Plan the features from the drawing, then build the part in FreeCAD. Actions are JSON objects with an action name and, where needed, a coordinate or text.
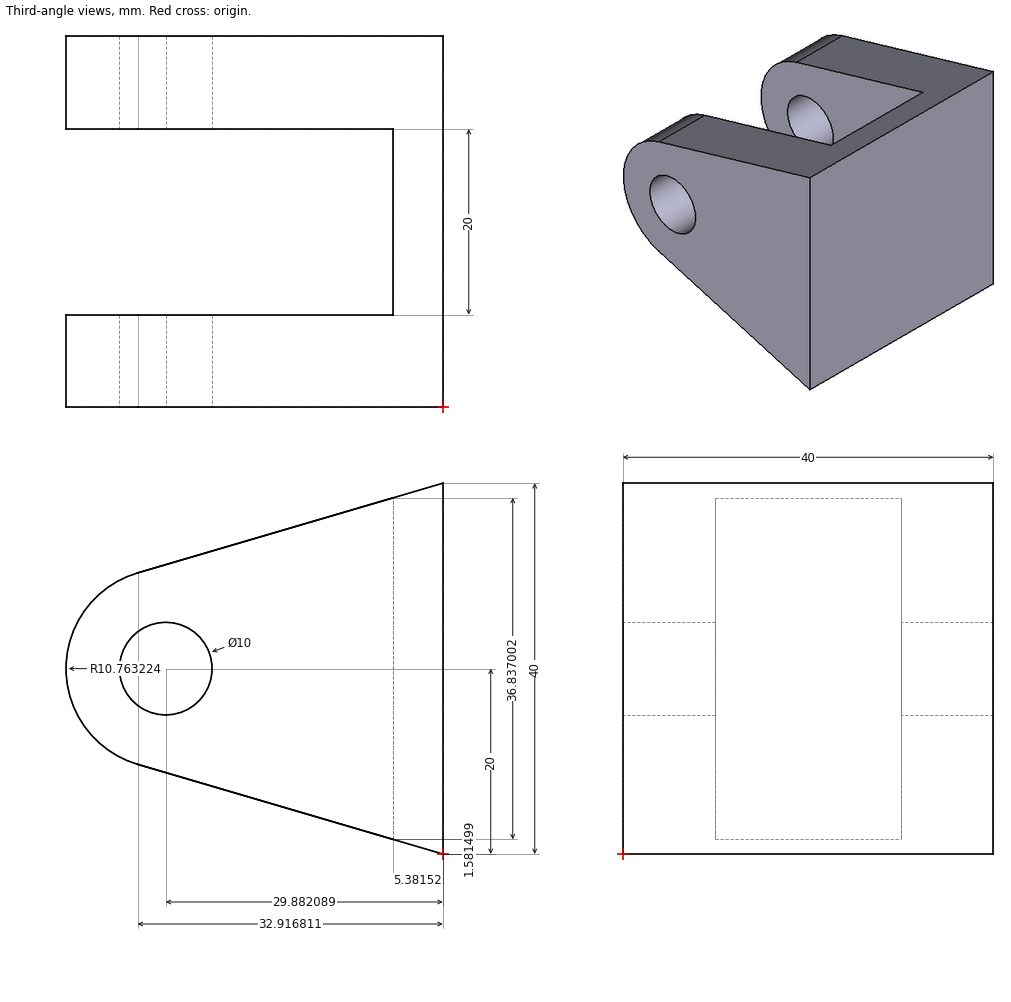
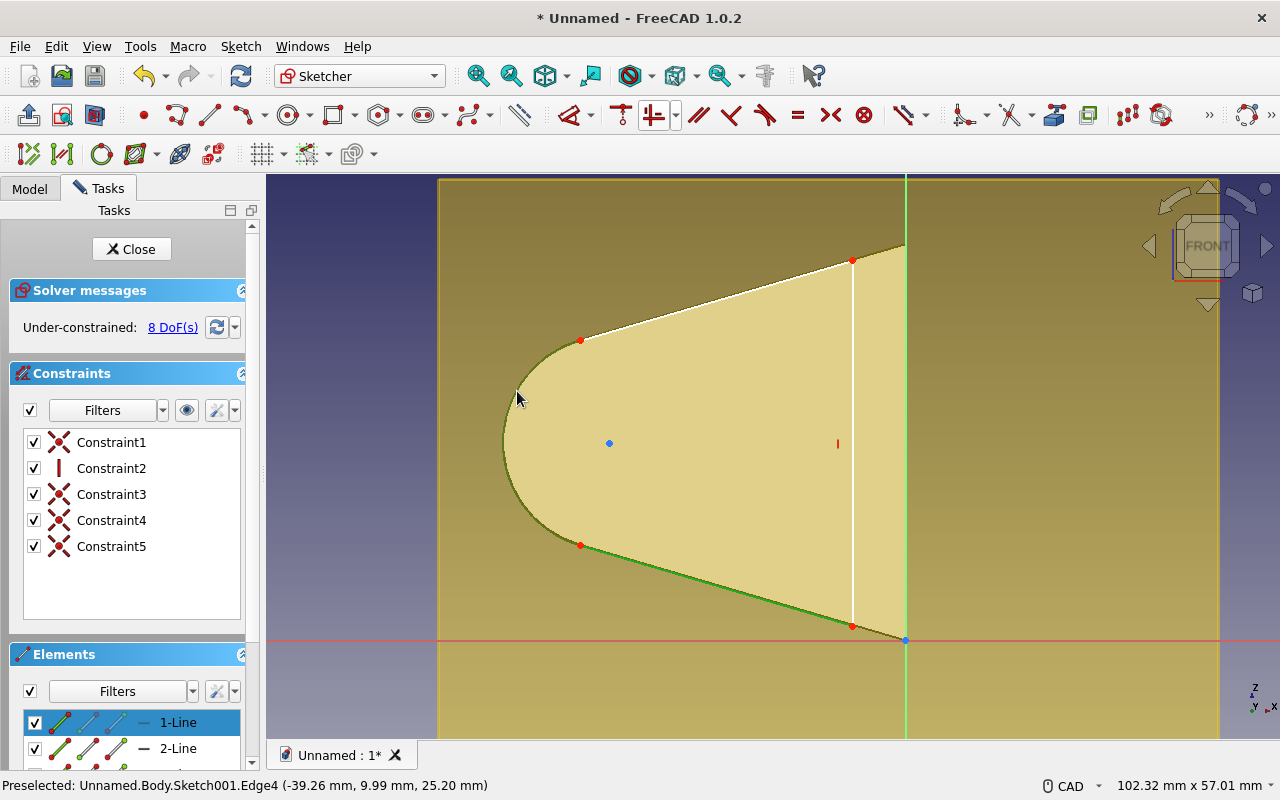
{"action": "left_click", "coordinate": [765, 116]}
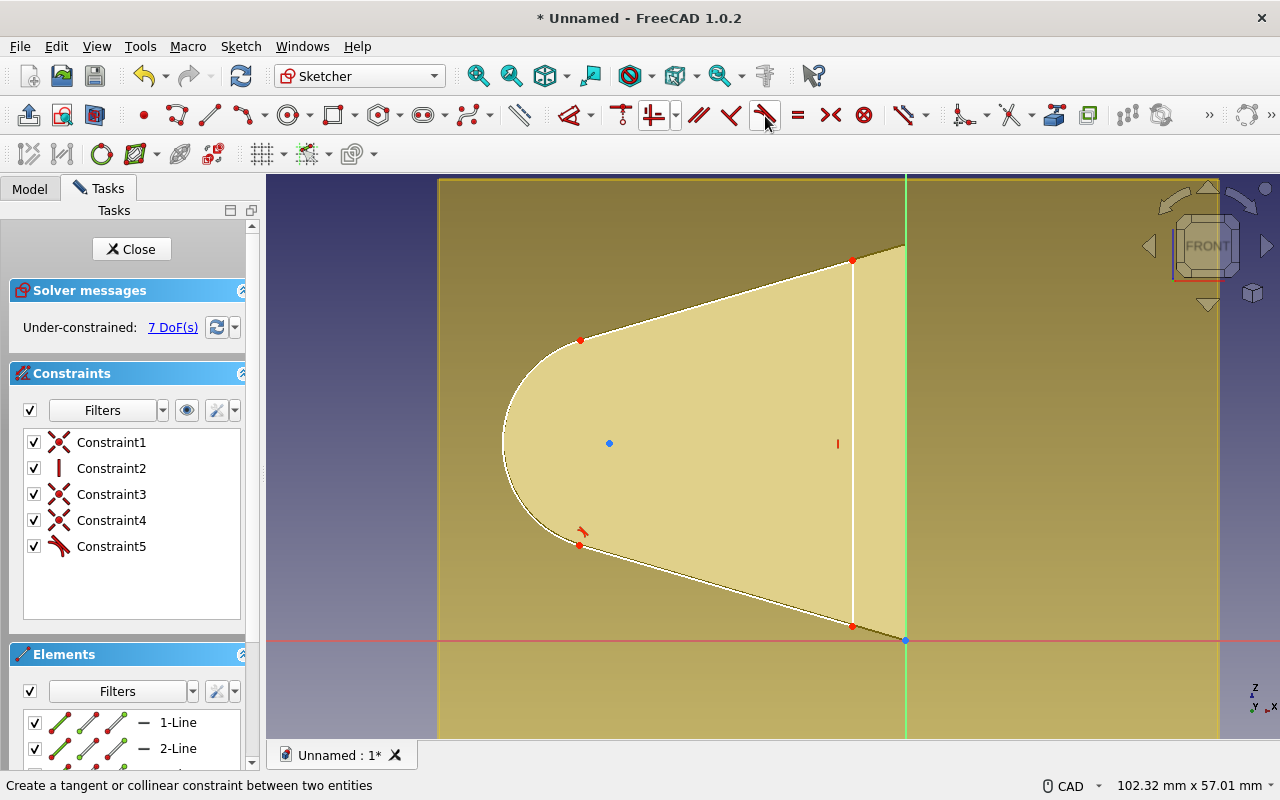
{"action": "left_click", "coordinate": [771, 285]}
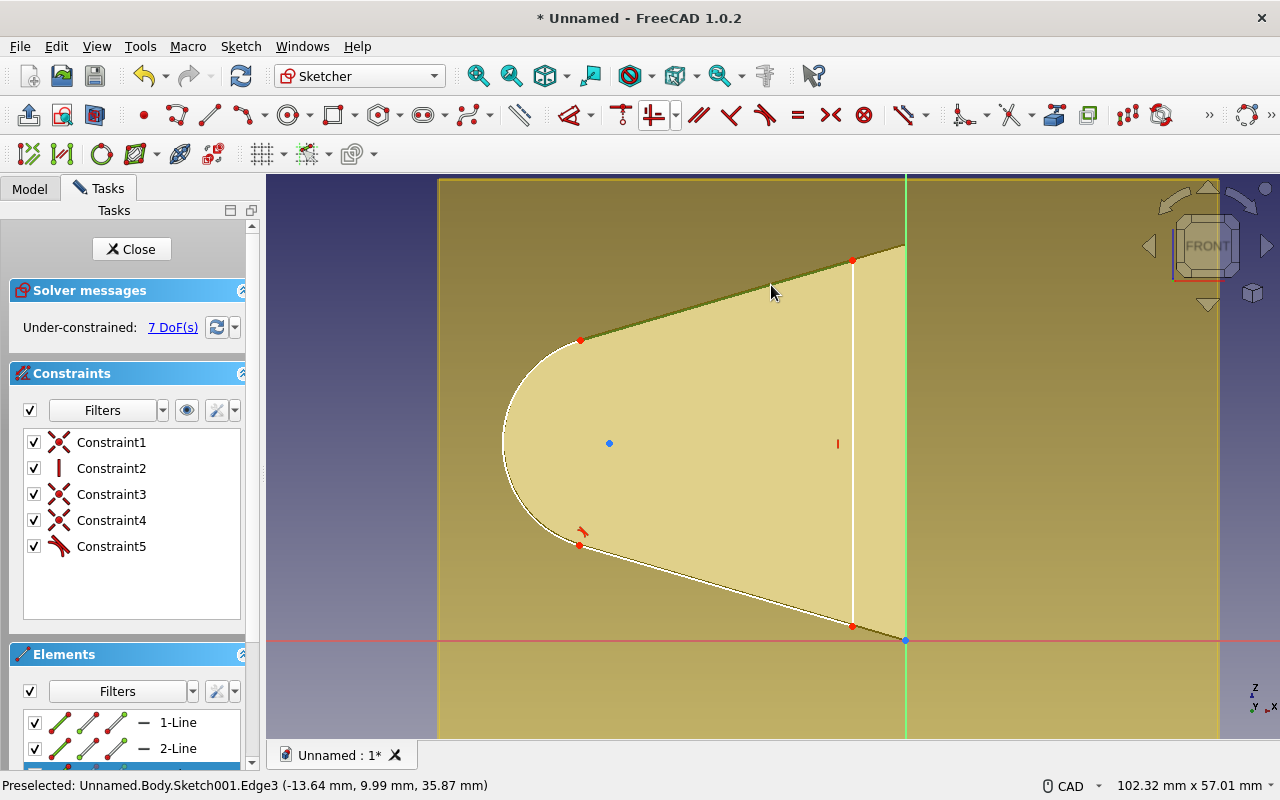
{"action": "left_click", "coordinate": [517, 391]}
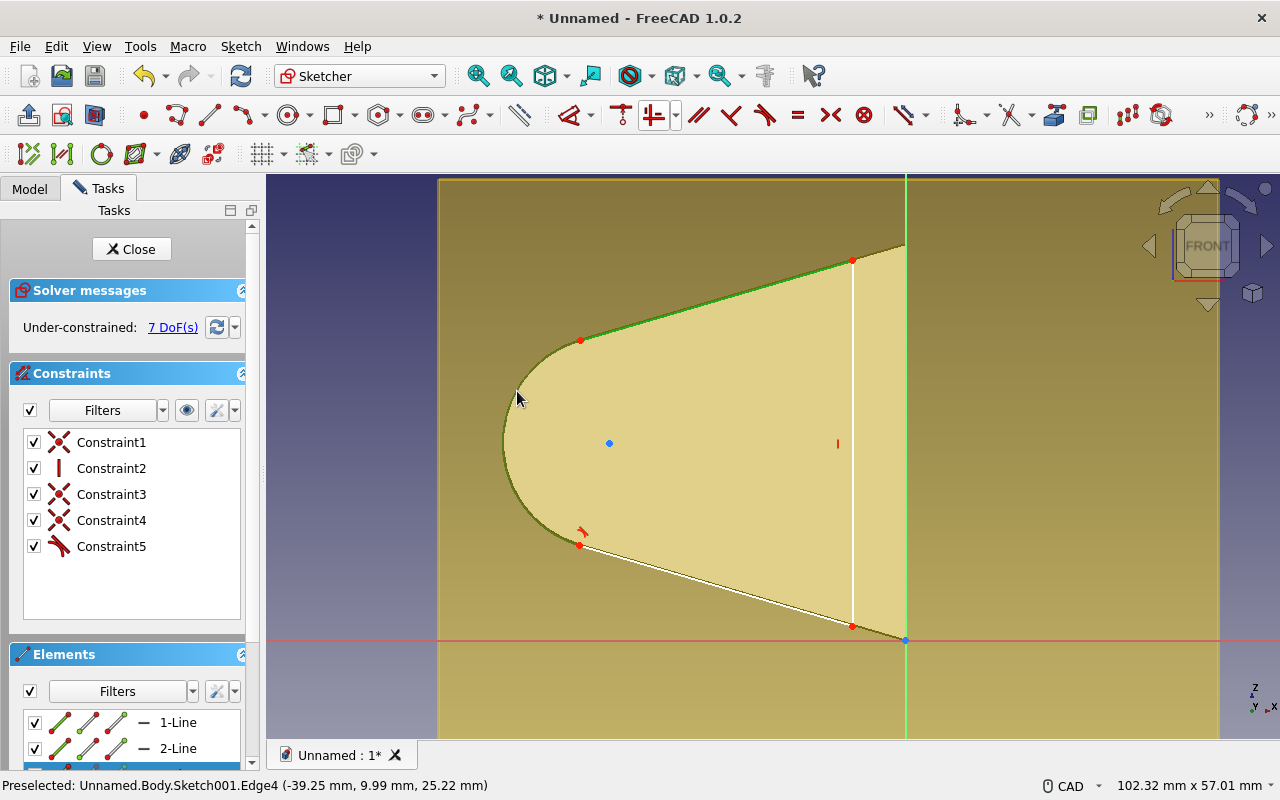
{"action": "left_click", "coordinate": [765, 116]}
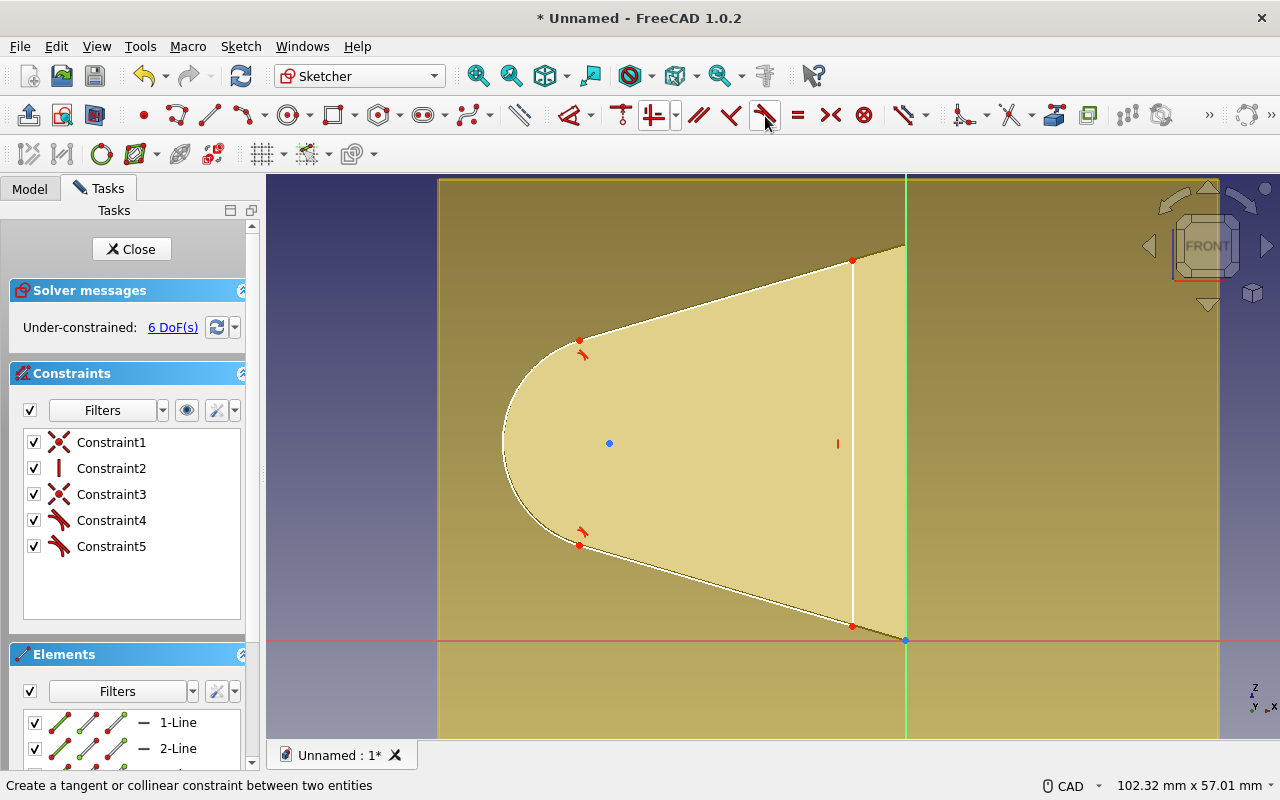
{"action": "left_click", "coordinate": [568, 116]}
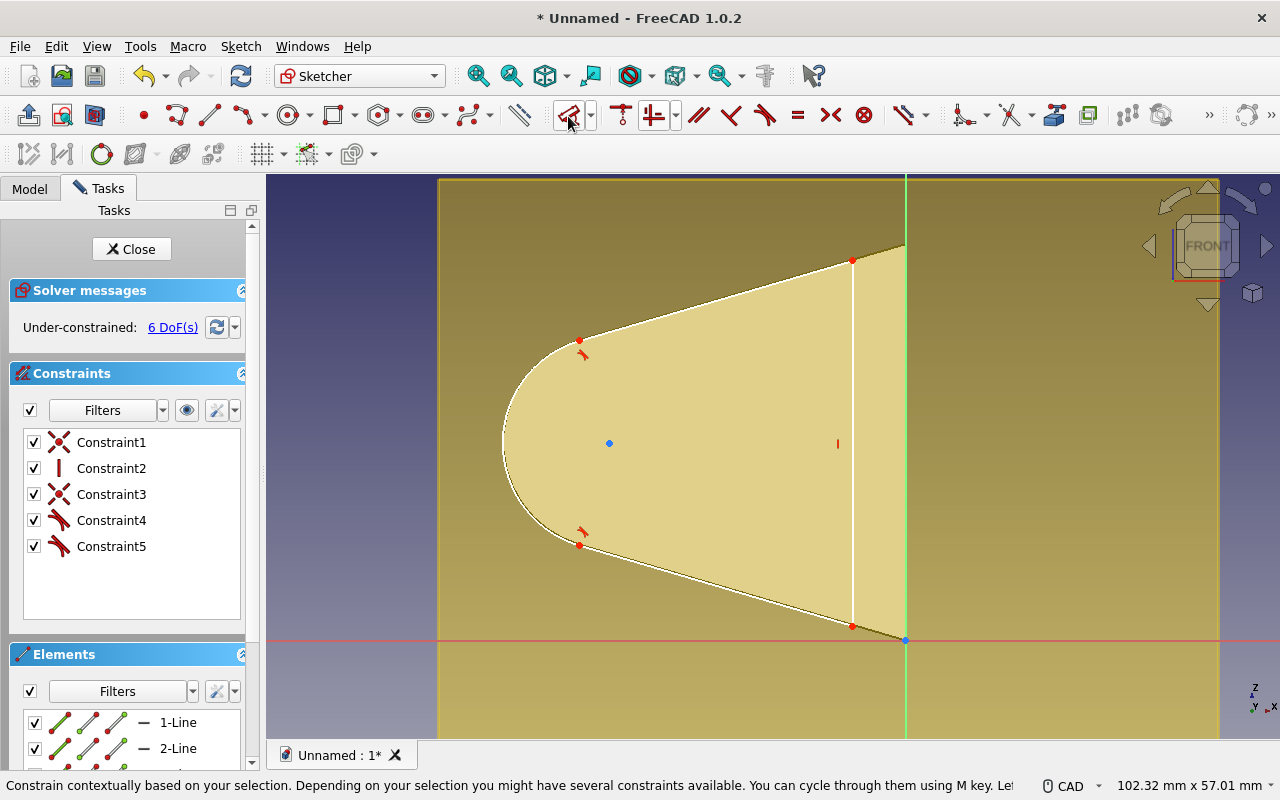
{"action": "left_click", "coordinate": [517, 391]}
{"action": "left_click", "coordinate": [489, 375]}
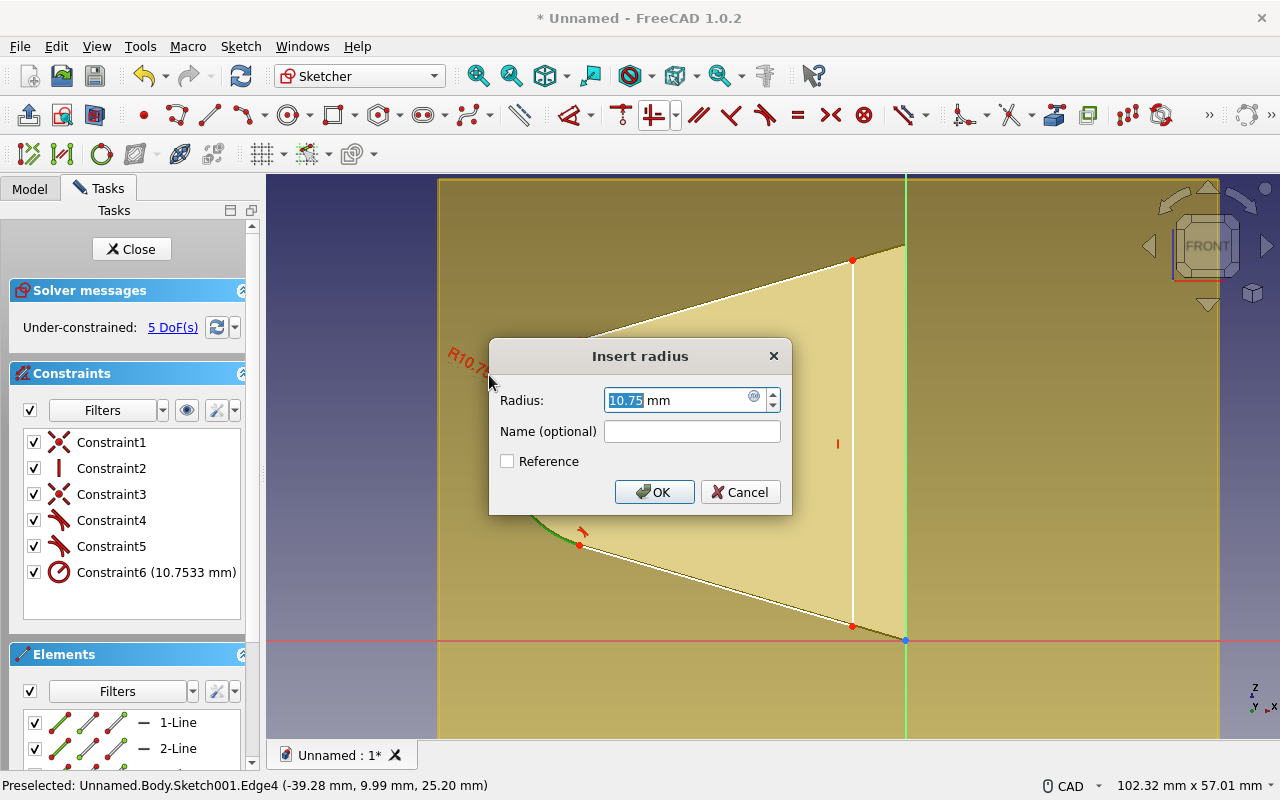
{"action": "type", "text": "10.763224"}
{"action": "key", "text": "Return"}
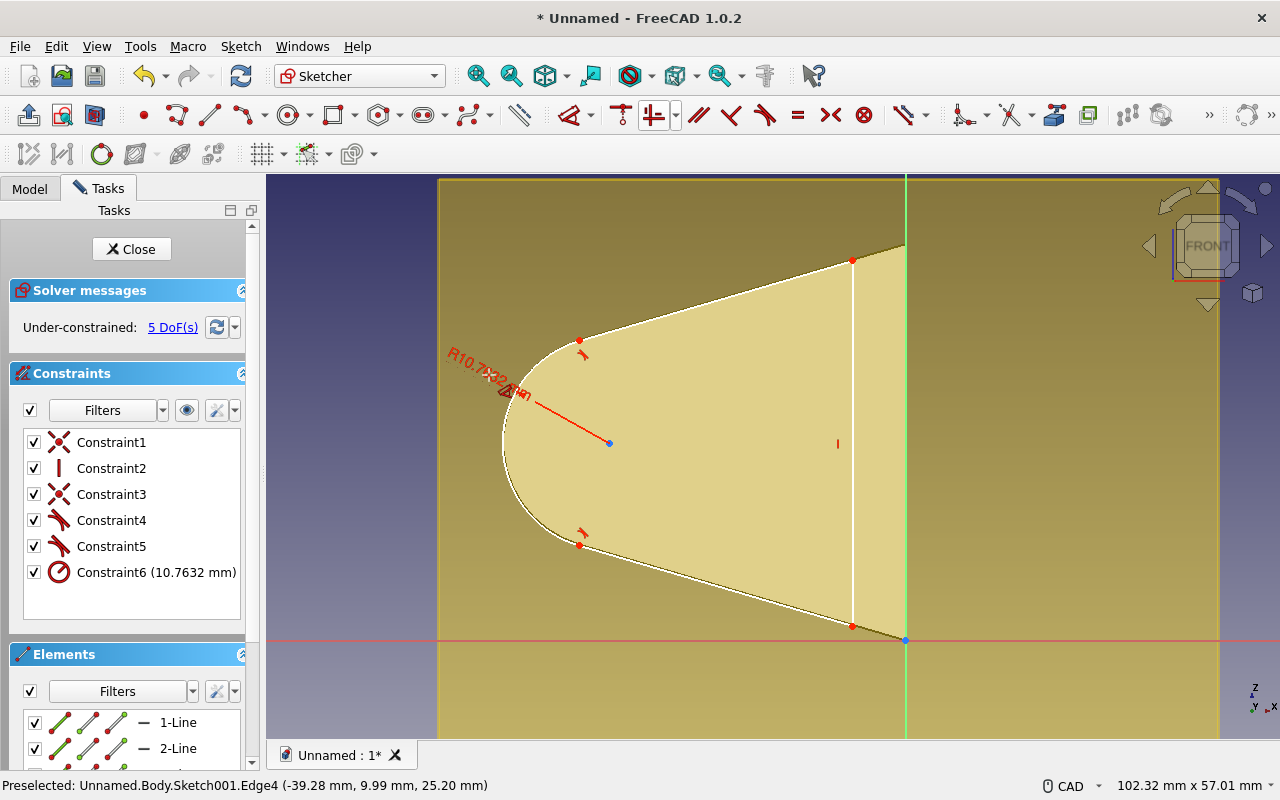
{"action": "left_click", "coordinate": [609, 443]}
{"action": "left_click", "coordinate": [940, 542]}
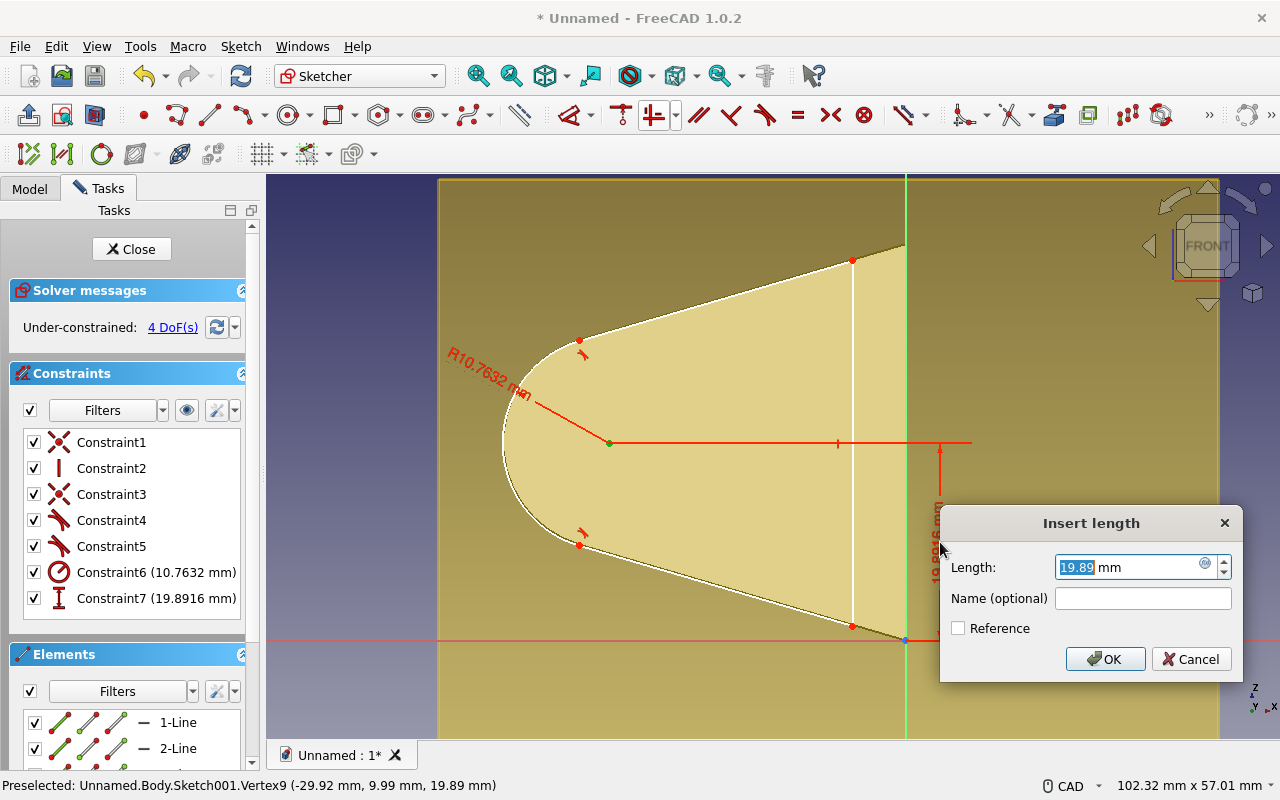
{"action": "type", "text": "20"}
{"action": "key", "text": "Return"}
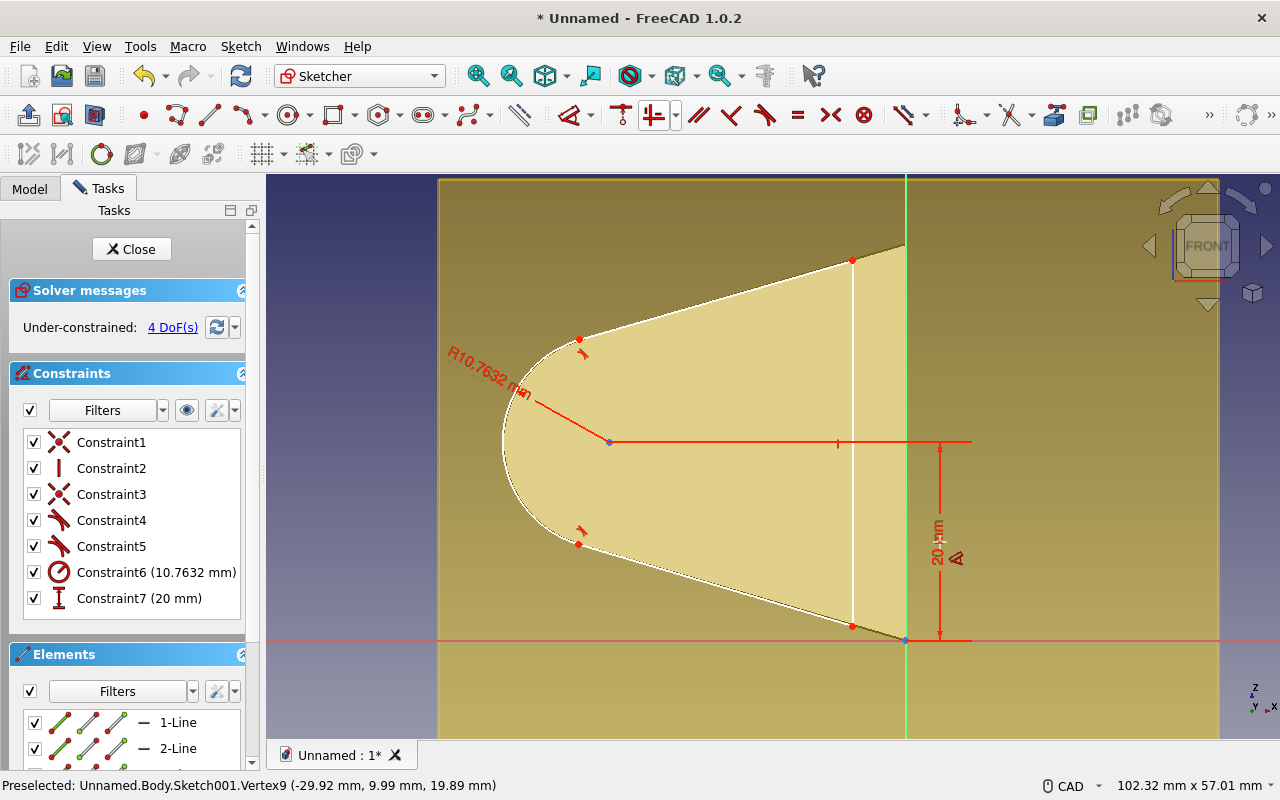
{"action": "left_click", "coordinate": [853, 626]}
{"action": "left_click", "coordinate": [879, 675]}